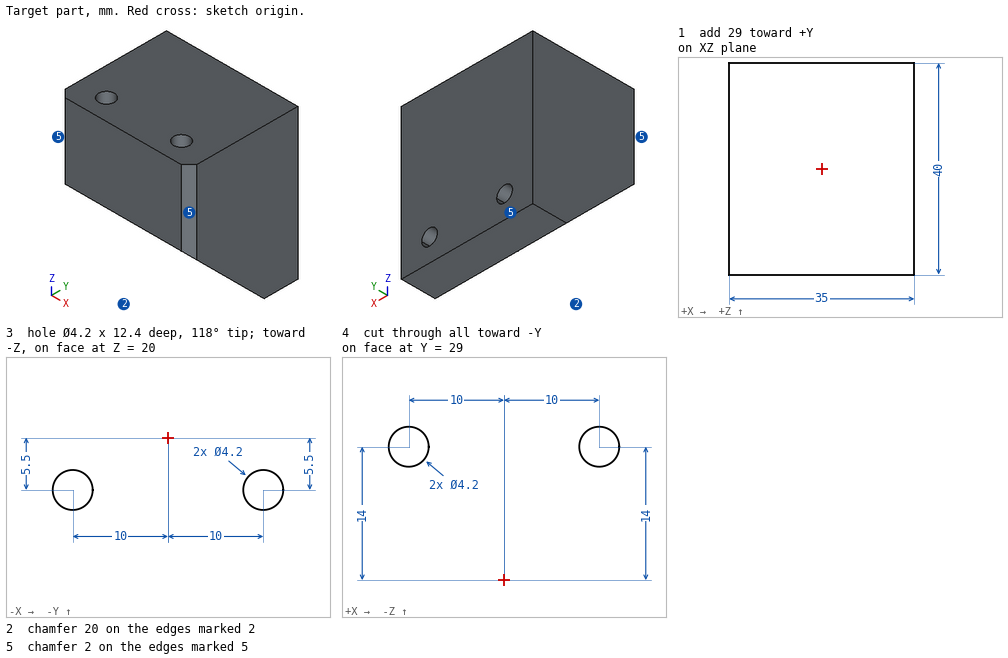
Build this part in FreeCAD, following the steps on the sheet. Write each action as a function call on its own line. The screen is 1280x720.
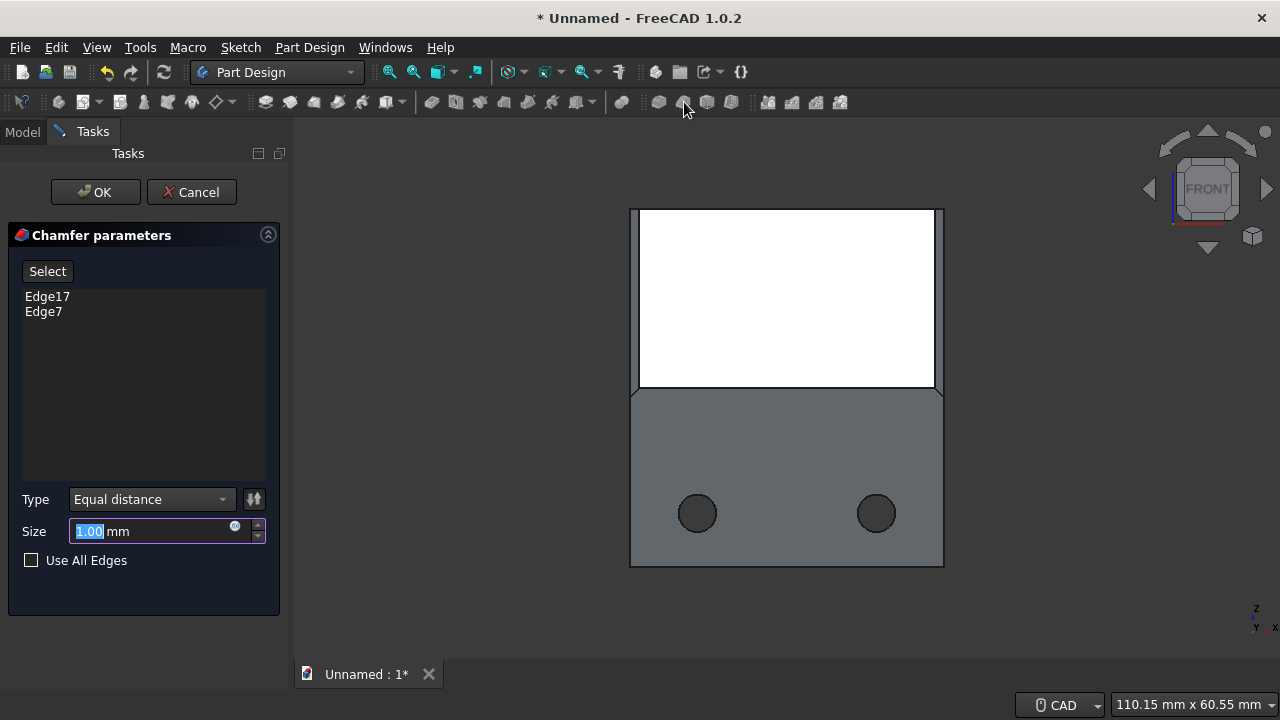
text(2)
key(Tab)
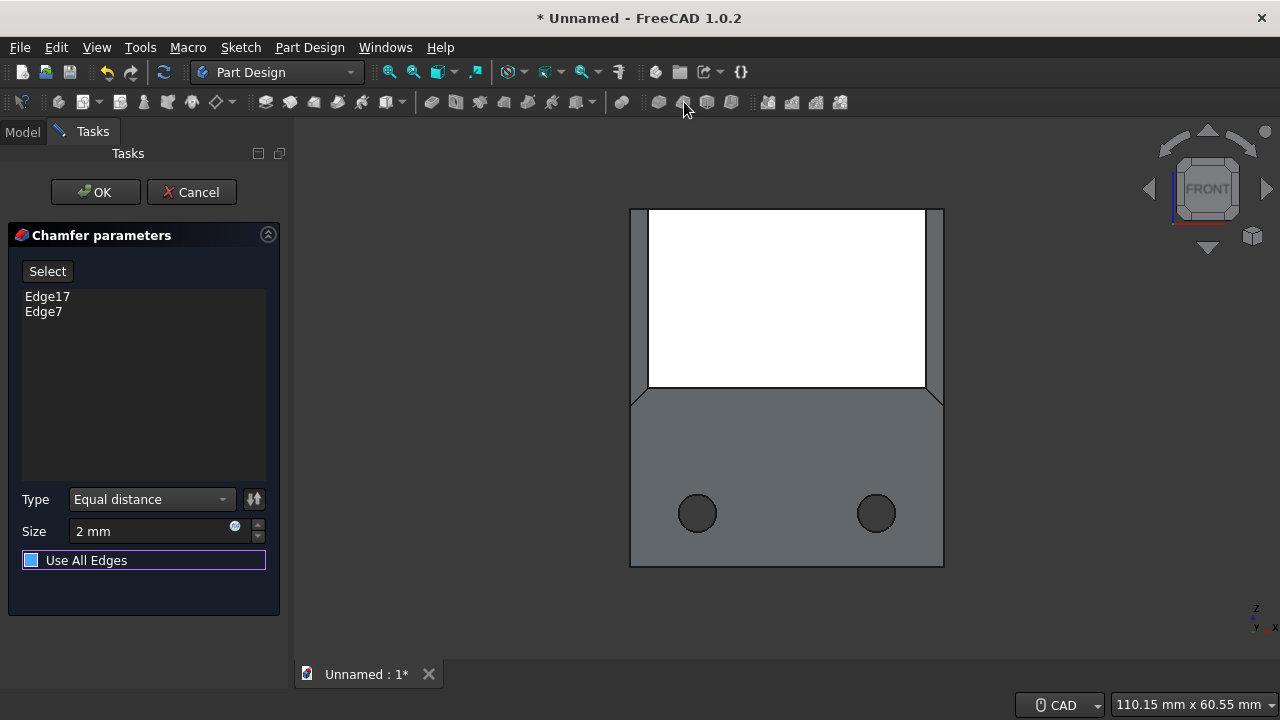
click(96, 192)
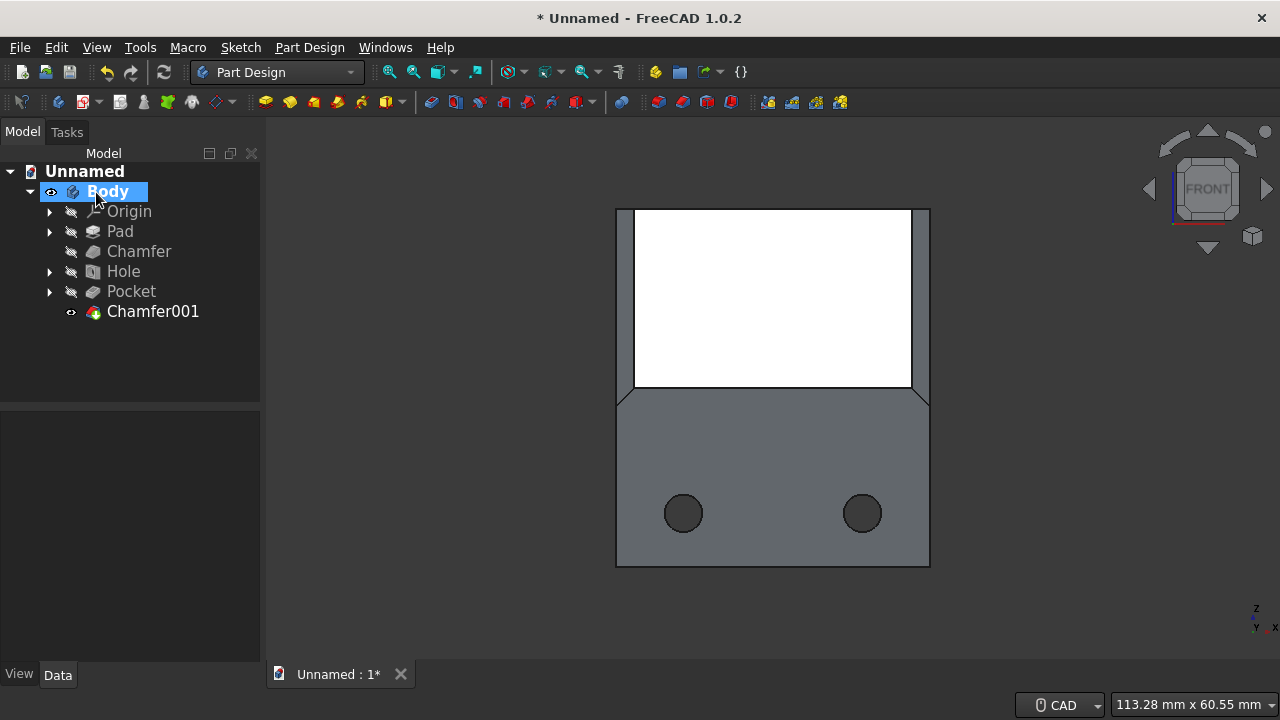
key(0)